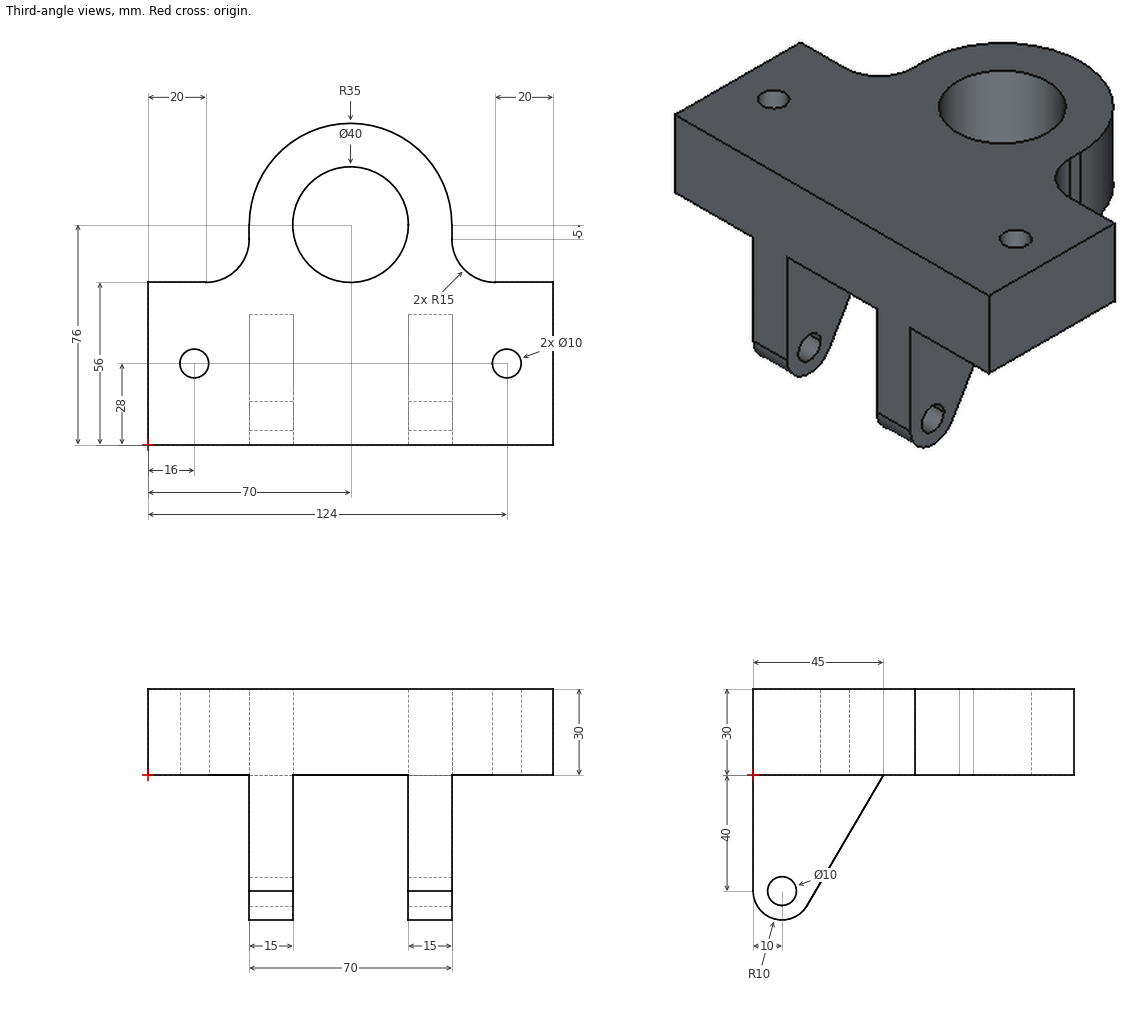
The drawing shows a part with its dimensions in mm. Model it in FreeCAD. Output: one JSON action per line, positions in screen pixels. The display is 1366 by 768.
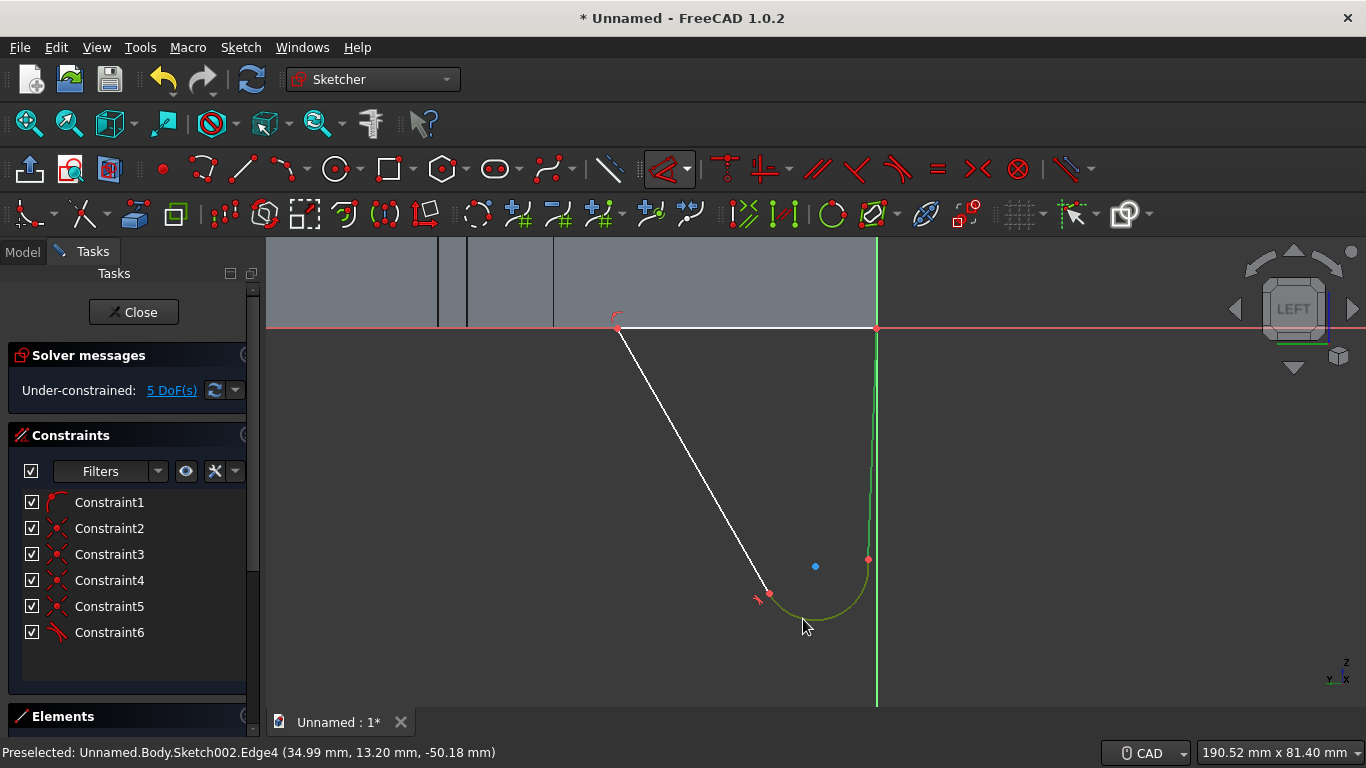
{"action": "left_click", "coordinate": [898, 170]}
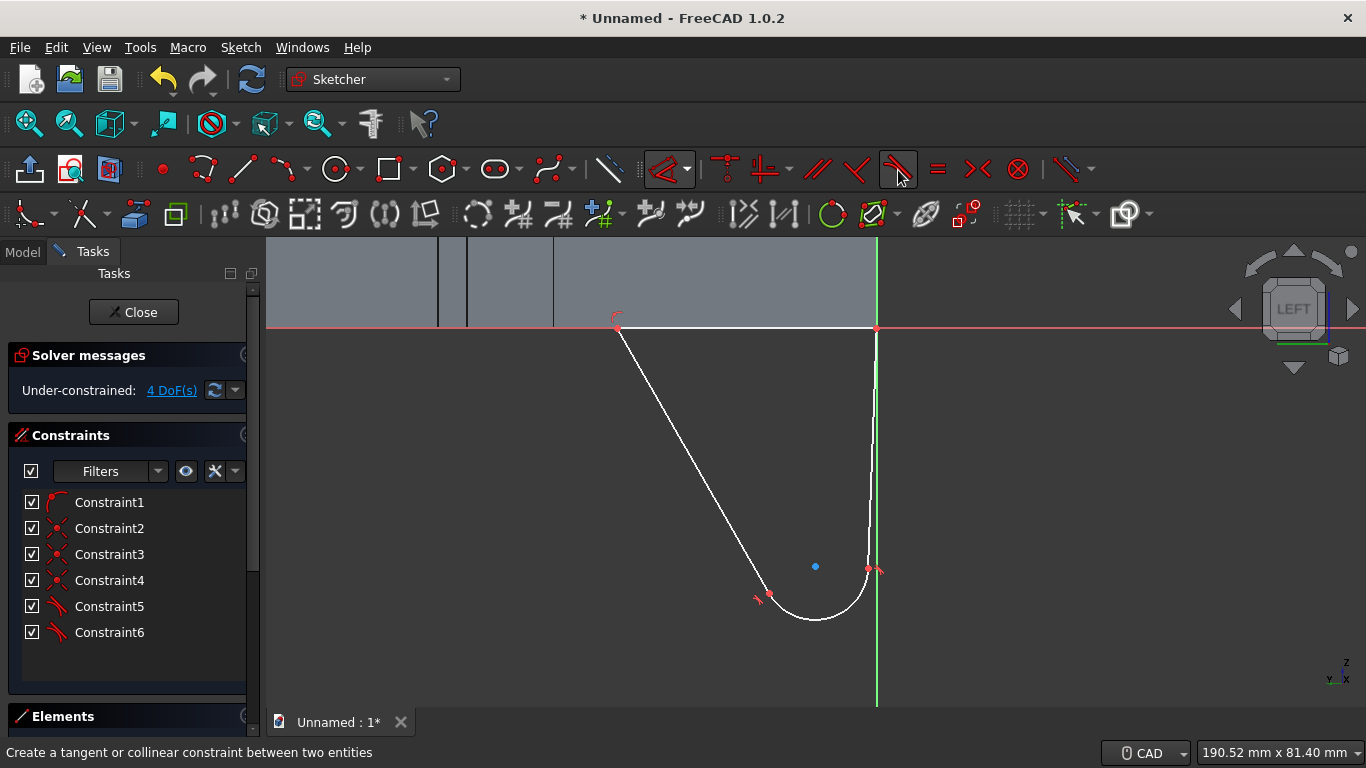
{"action": "left_click", "coordinate": [874, 400]}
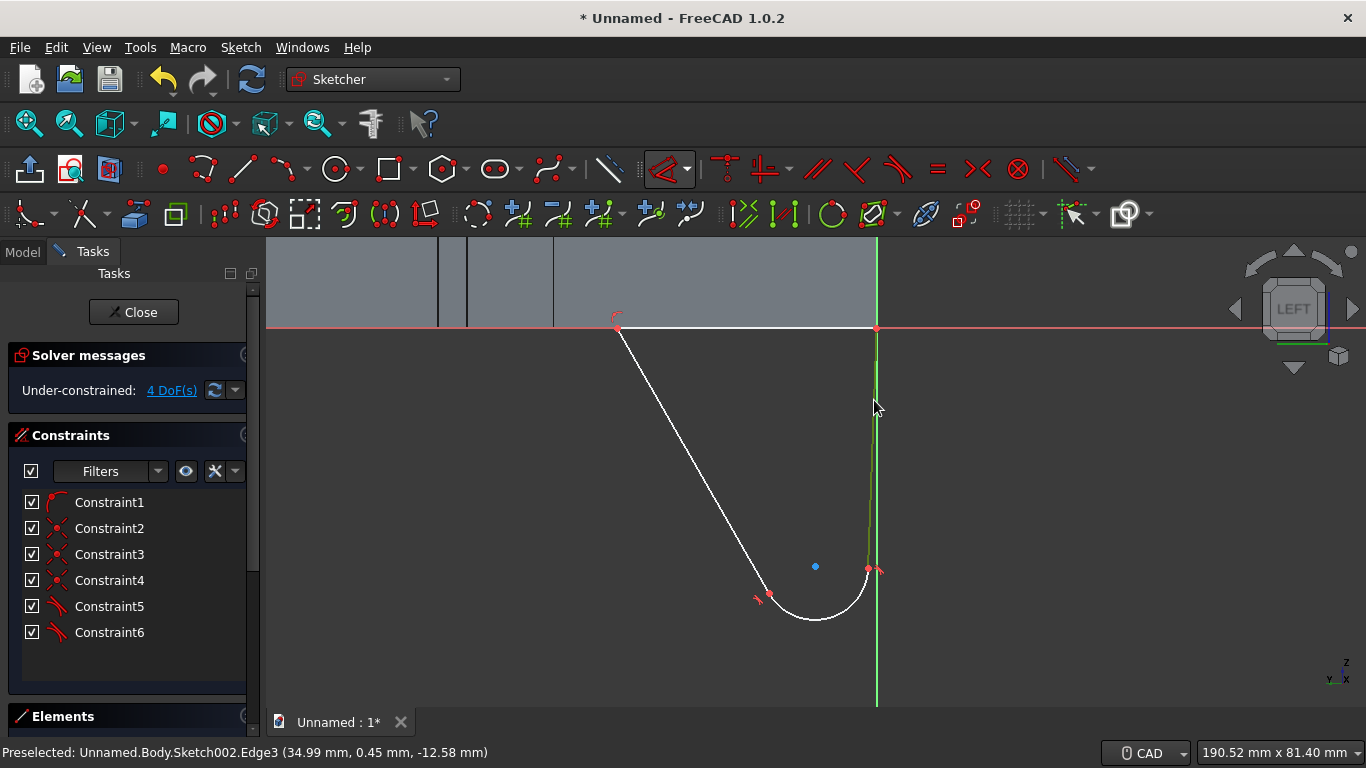
{"action": "key", "text": "v"}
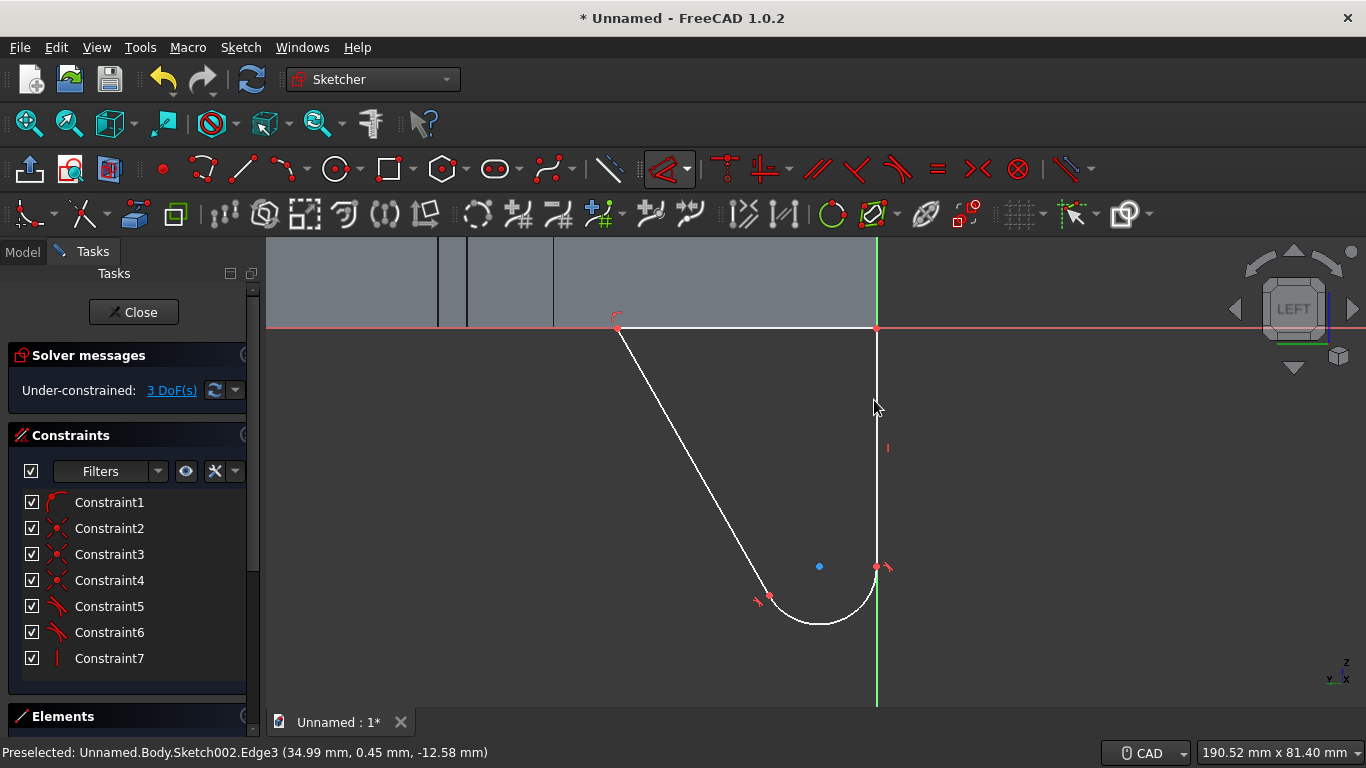
{"action": "left_click", "coordinate": [804, 622]}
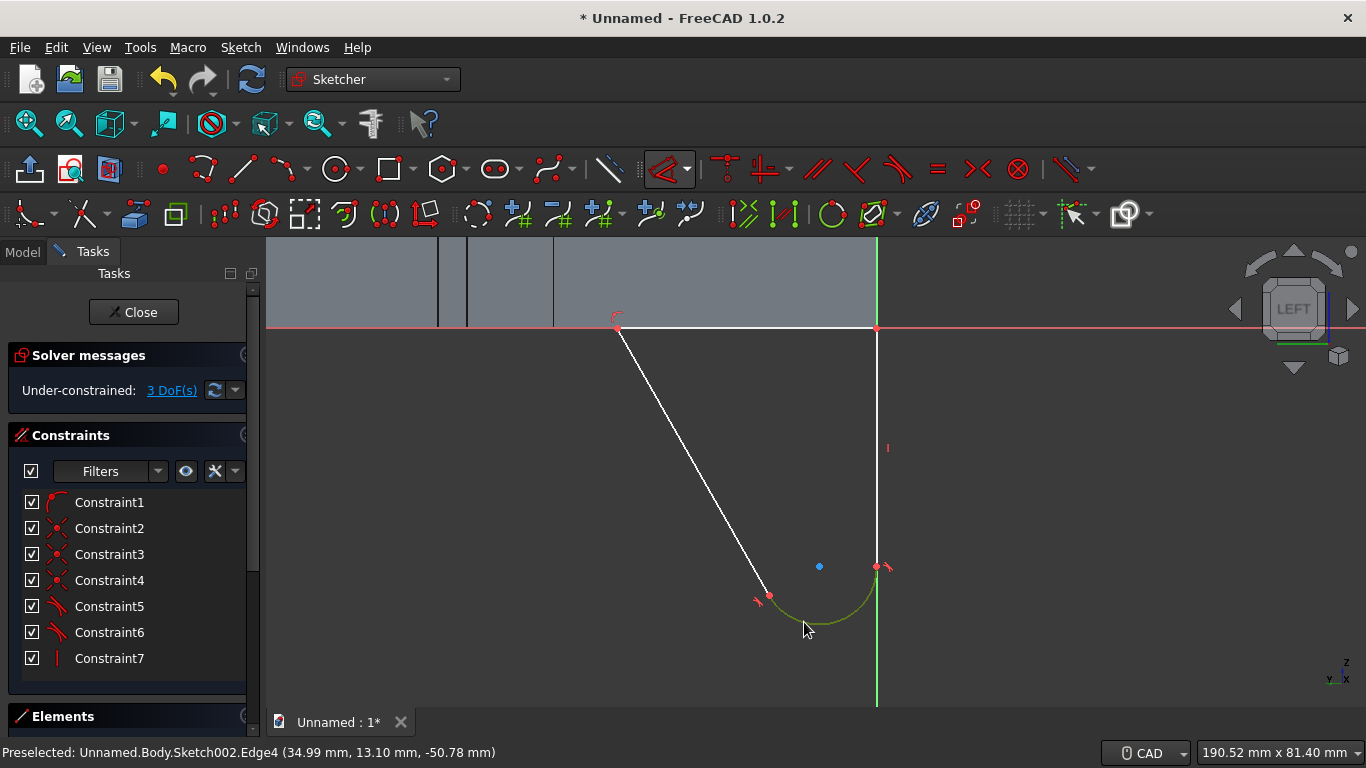
{"action": "left_click", "coordinate": [690, 170]}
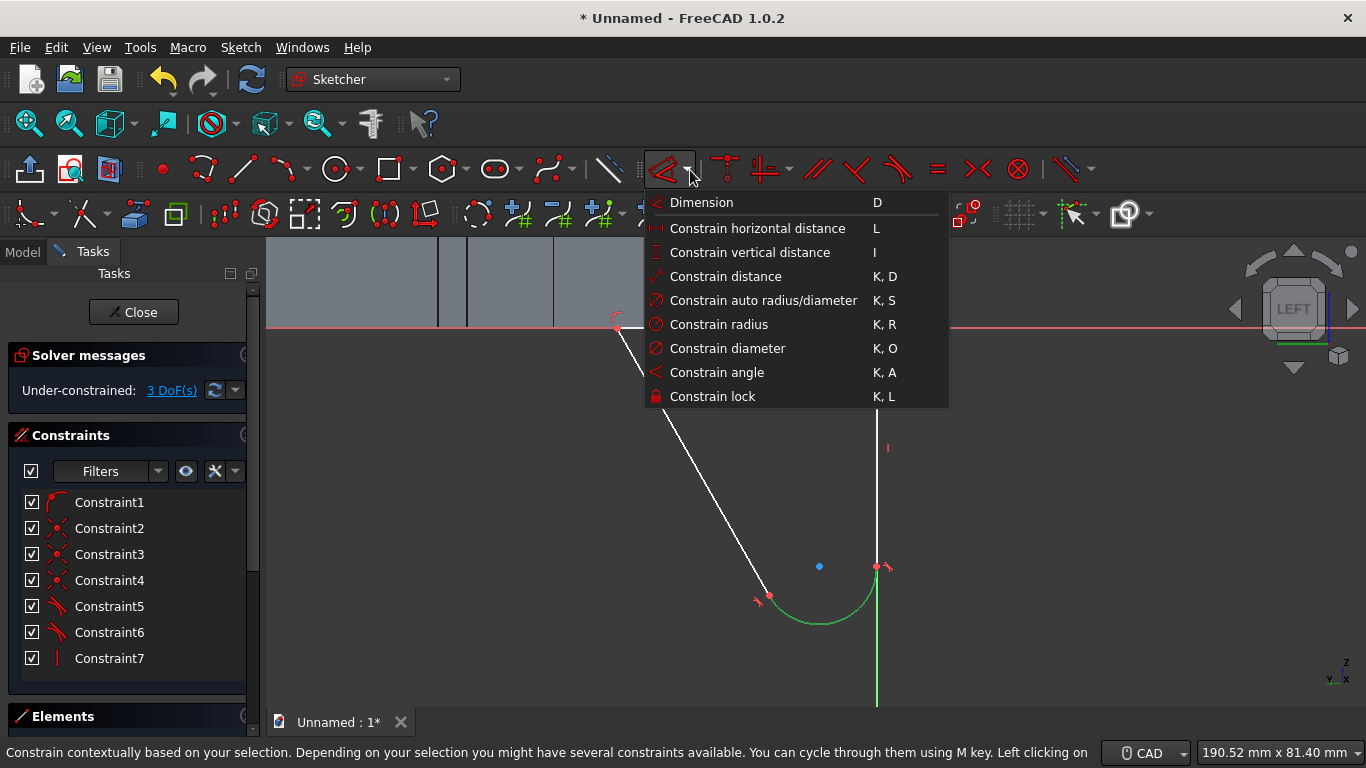
{"action": "left_click", "coordinate": [797, 324]}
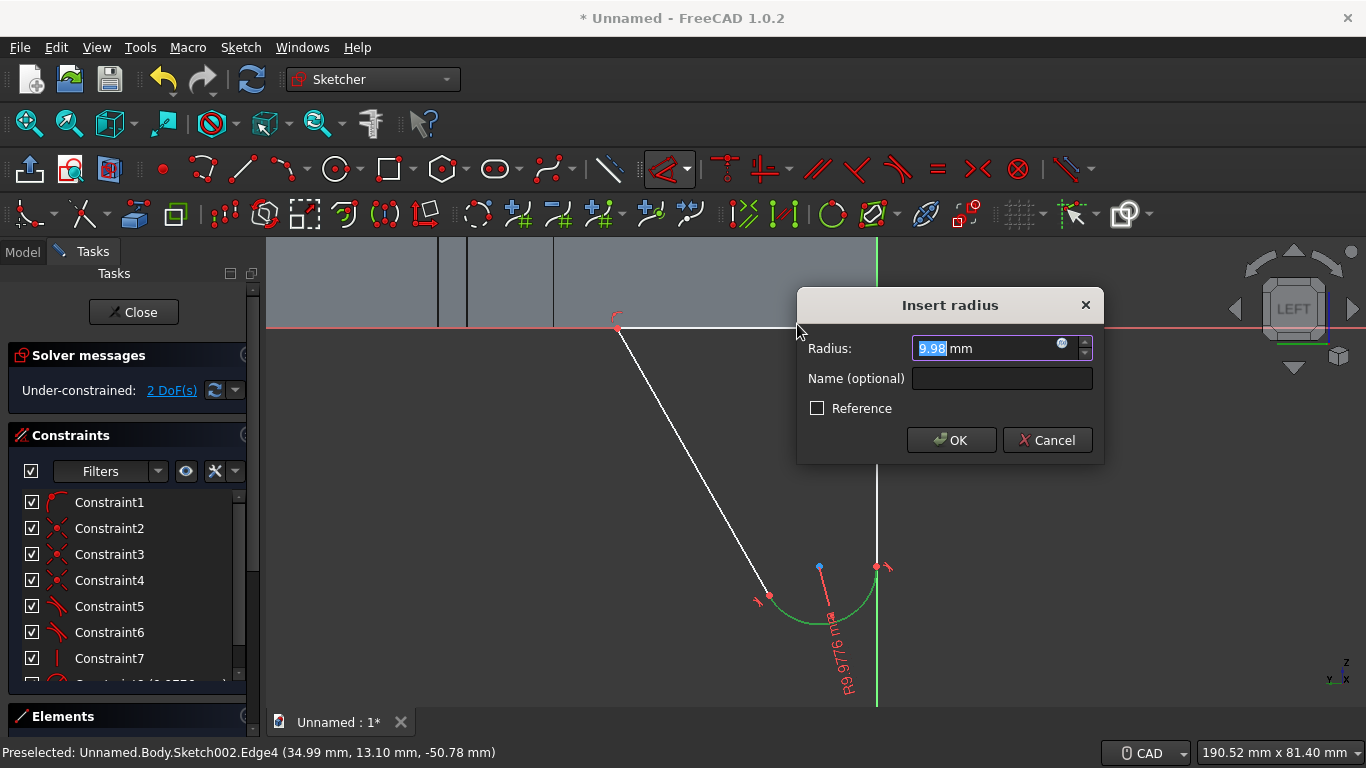
{"action": "type", "text": "10"}
{"action": "key", "text": "Return"}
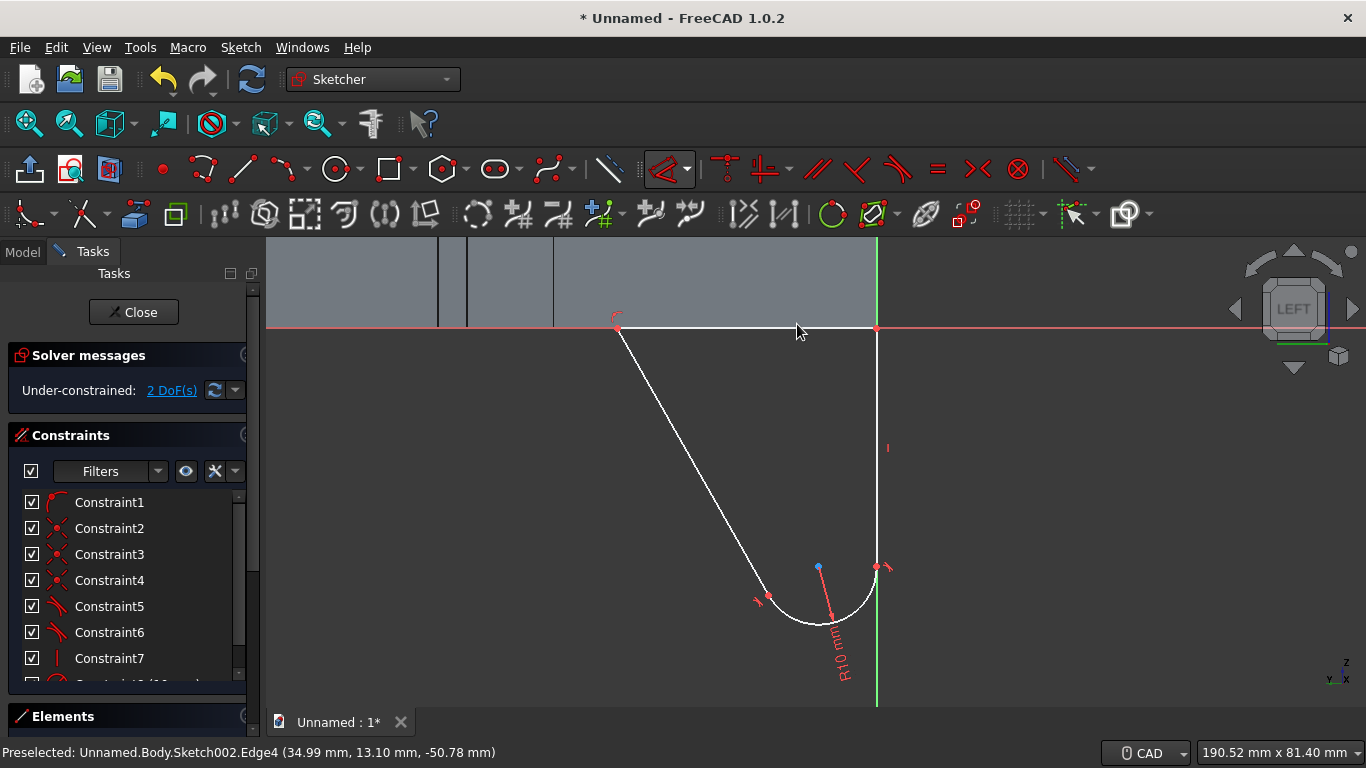
{"action": "left_click", "coordinate": [695, 328]}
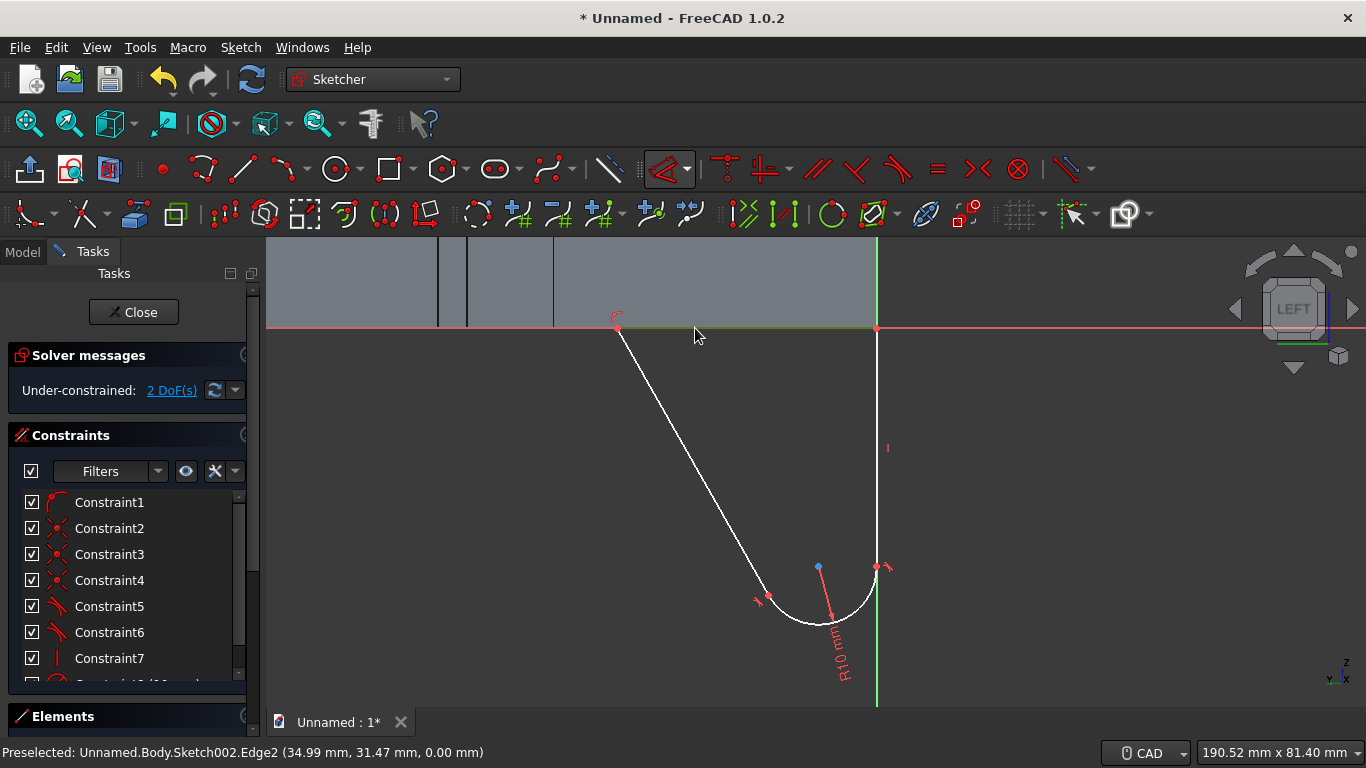
{"action": "left_click", "coordinate": [690, 170]}